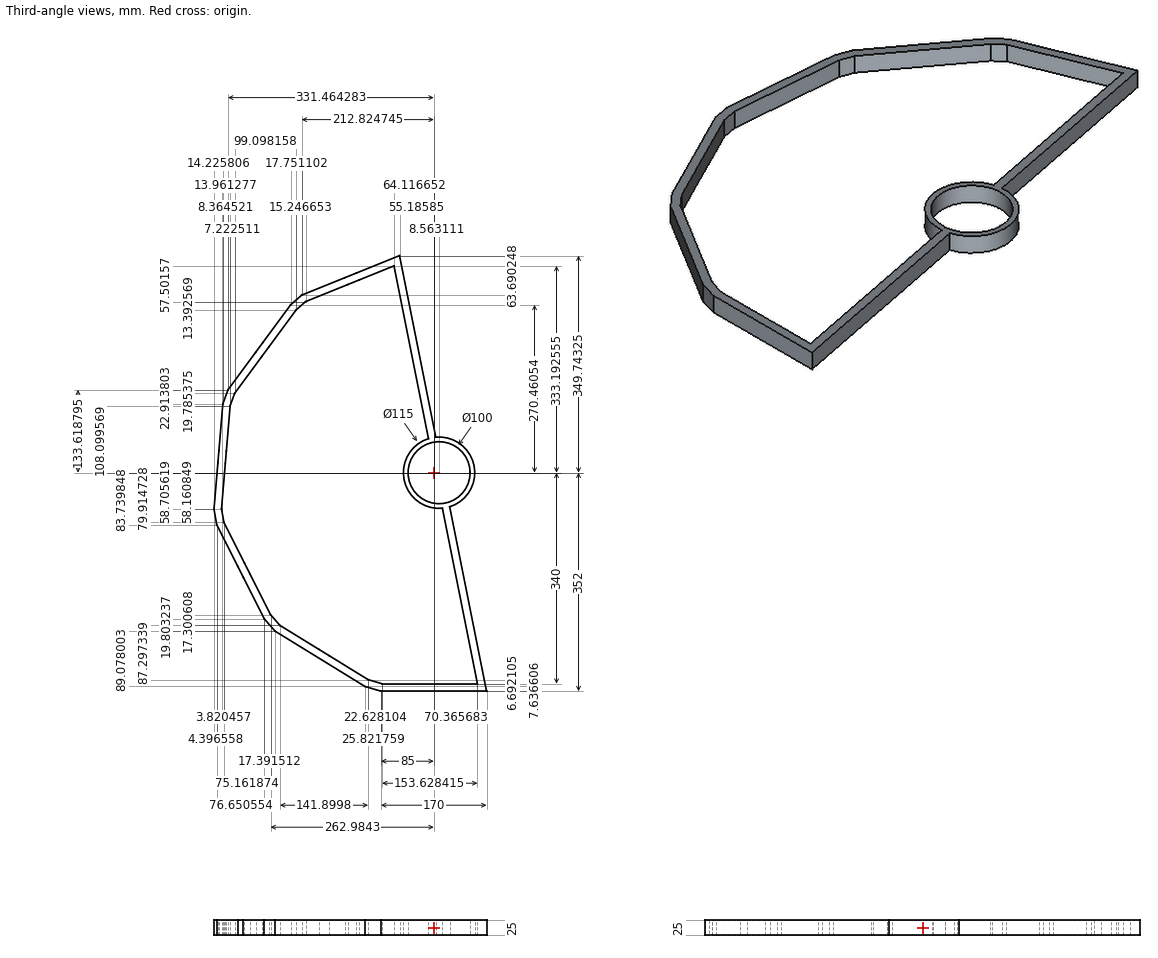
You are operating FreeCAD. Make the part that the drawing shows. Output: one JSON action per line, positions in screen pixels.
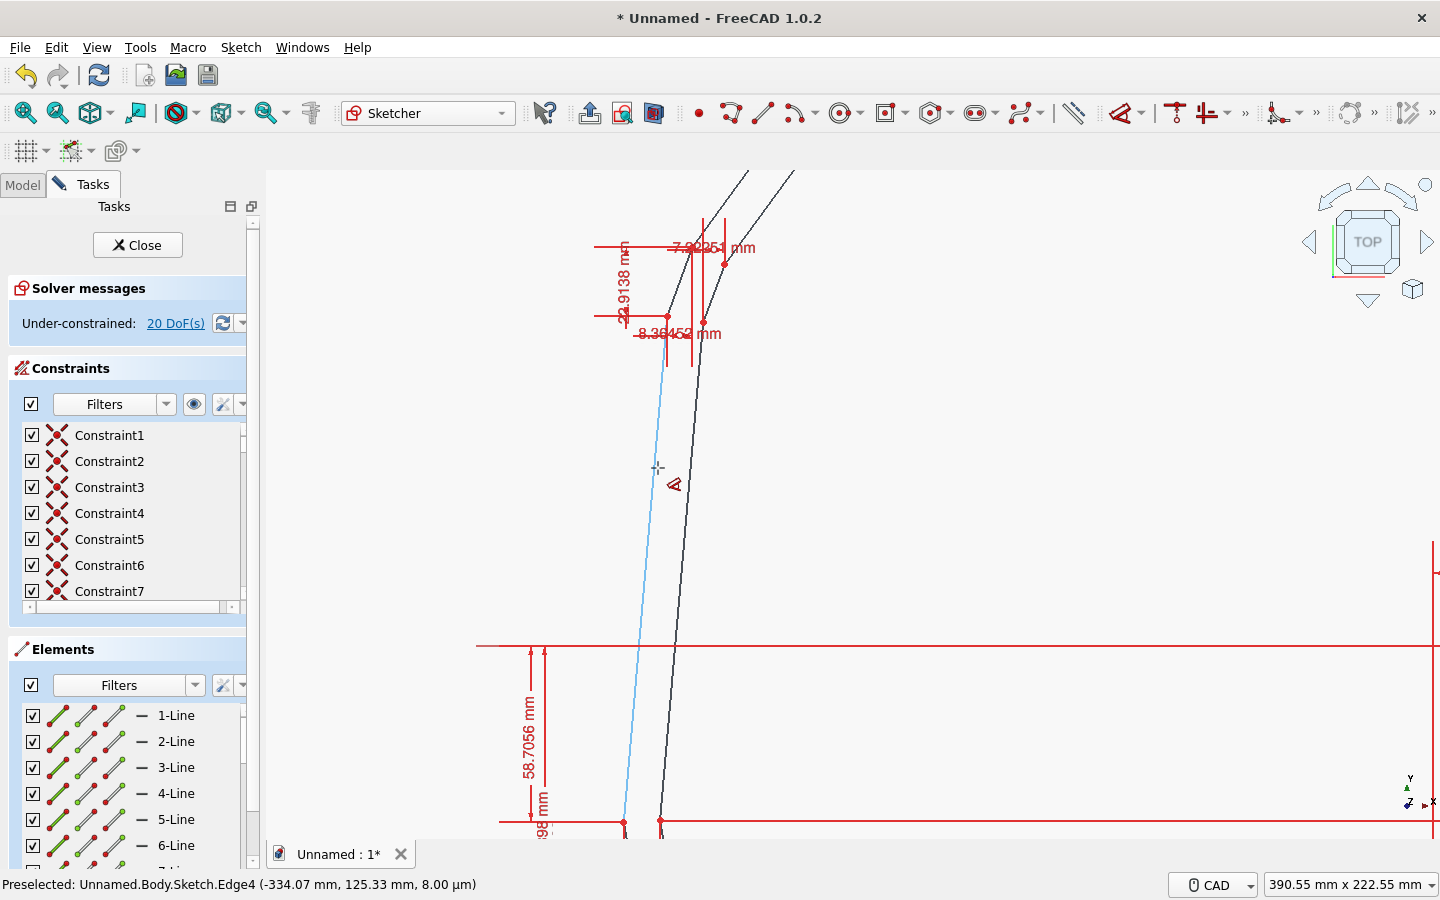
{"action": "left_click", "coordinate": [654, 468]}
{"action": "left_click", "coordinate": [636, 258]}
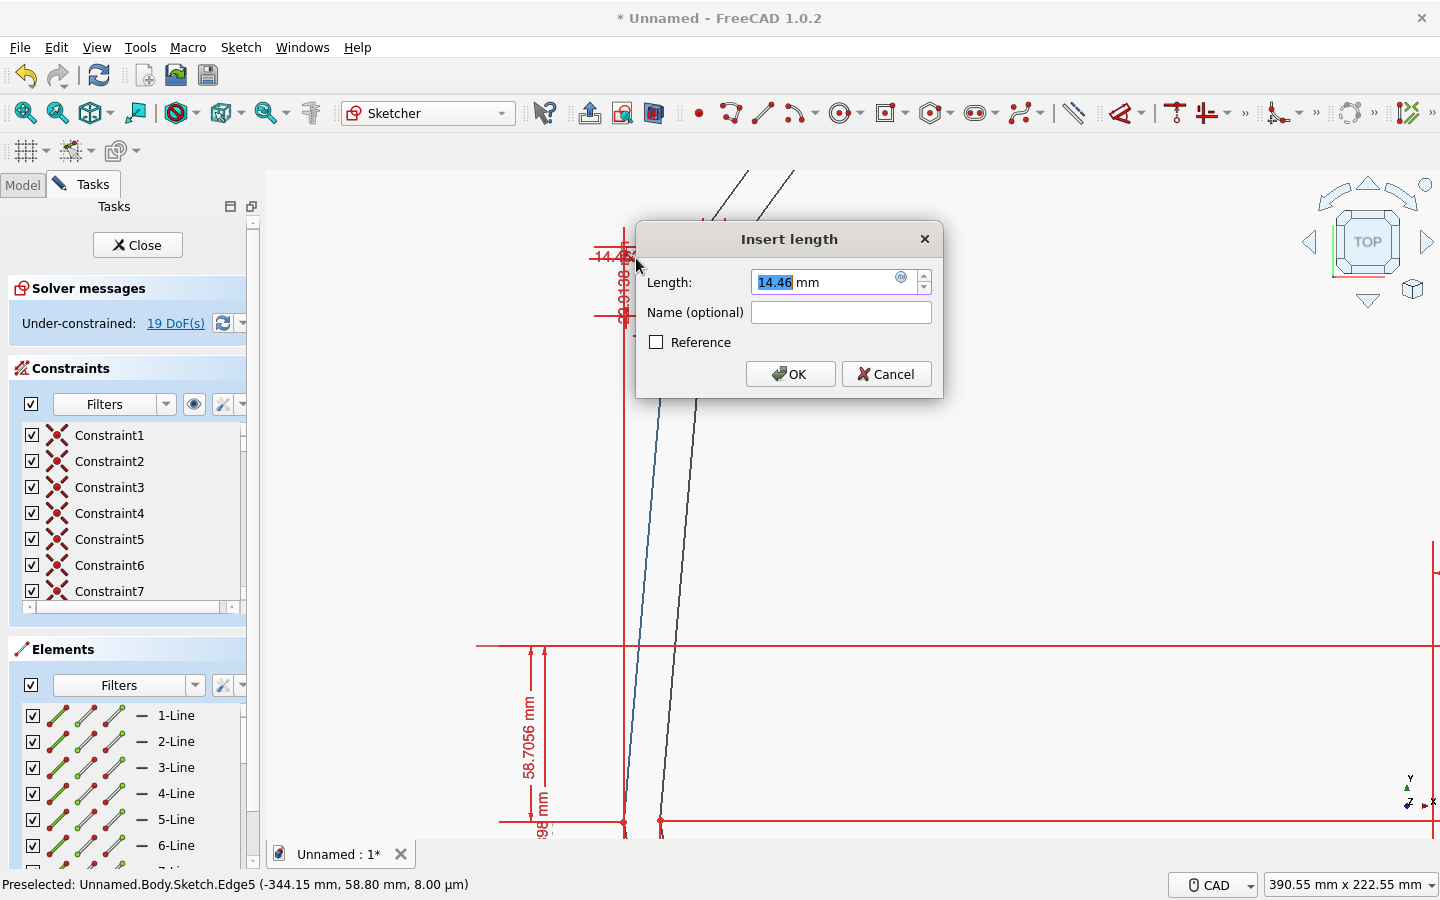
{"action": "type", "text": "14.225806"}
{"action": "key", "text": "Return"}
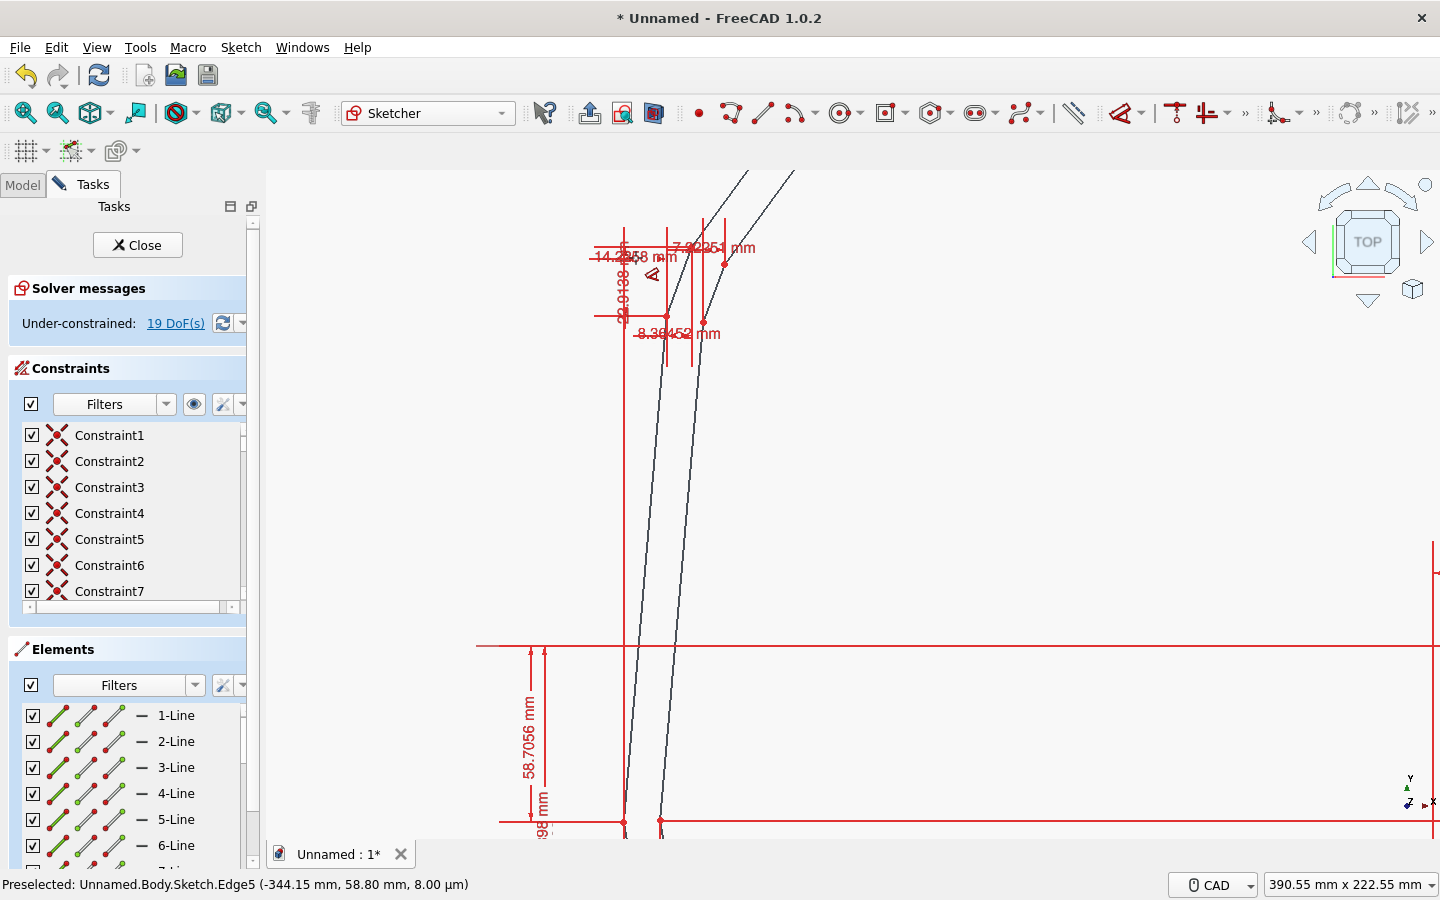
{"action": "scroll", "coordinate": [658, 468], "scroll_direction": "down", "scroll_amount": 8}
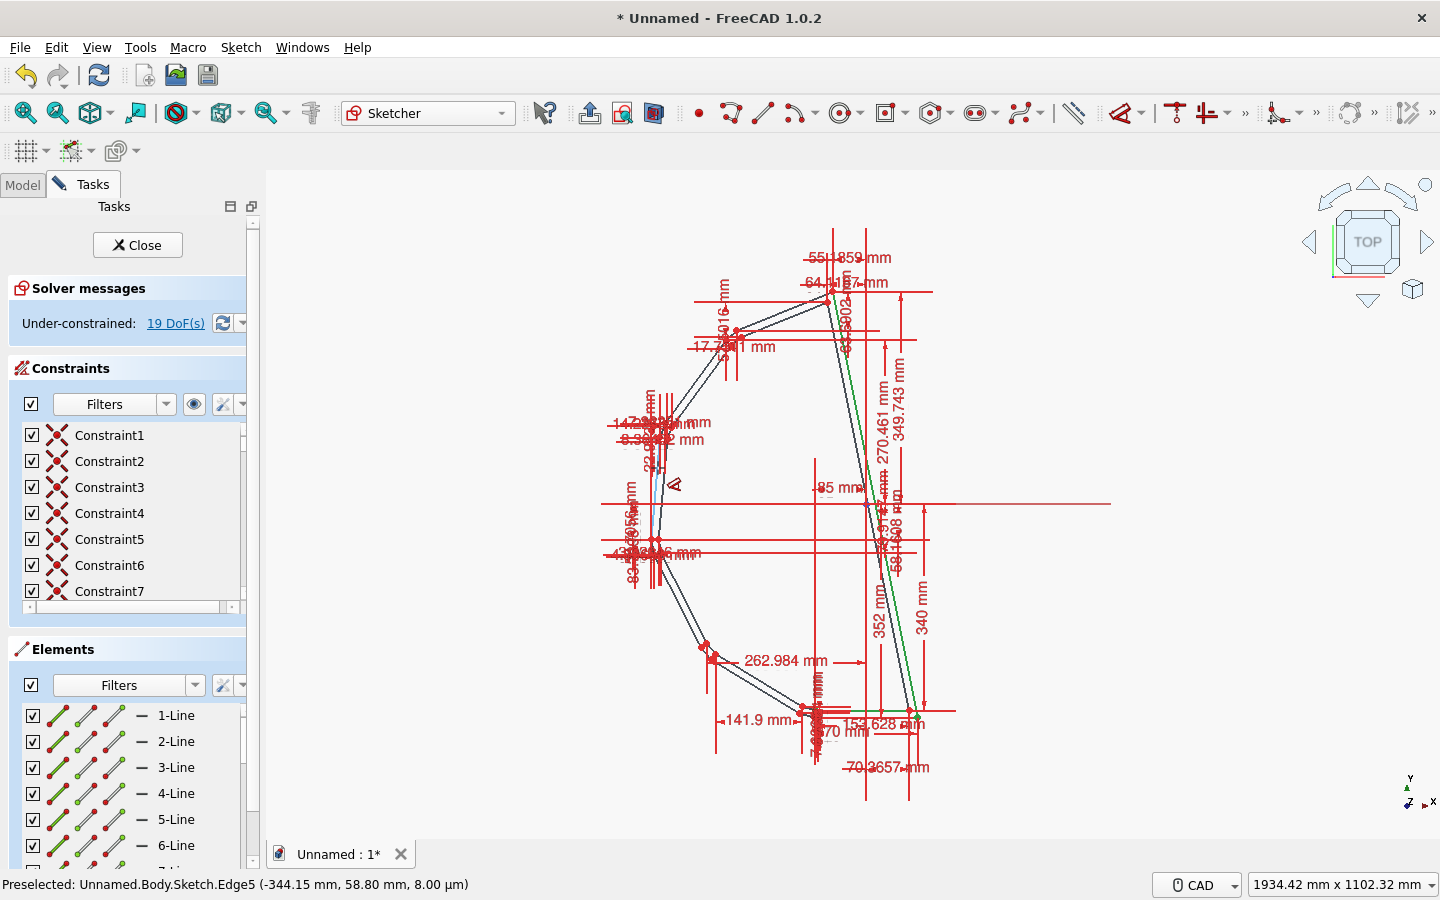
{"action": "scroll", "coordinate": [668, 583], "scroll_direction": "up", "scroll_amount": 4}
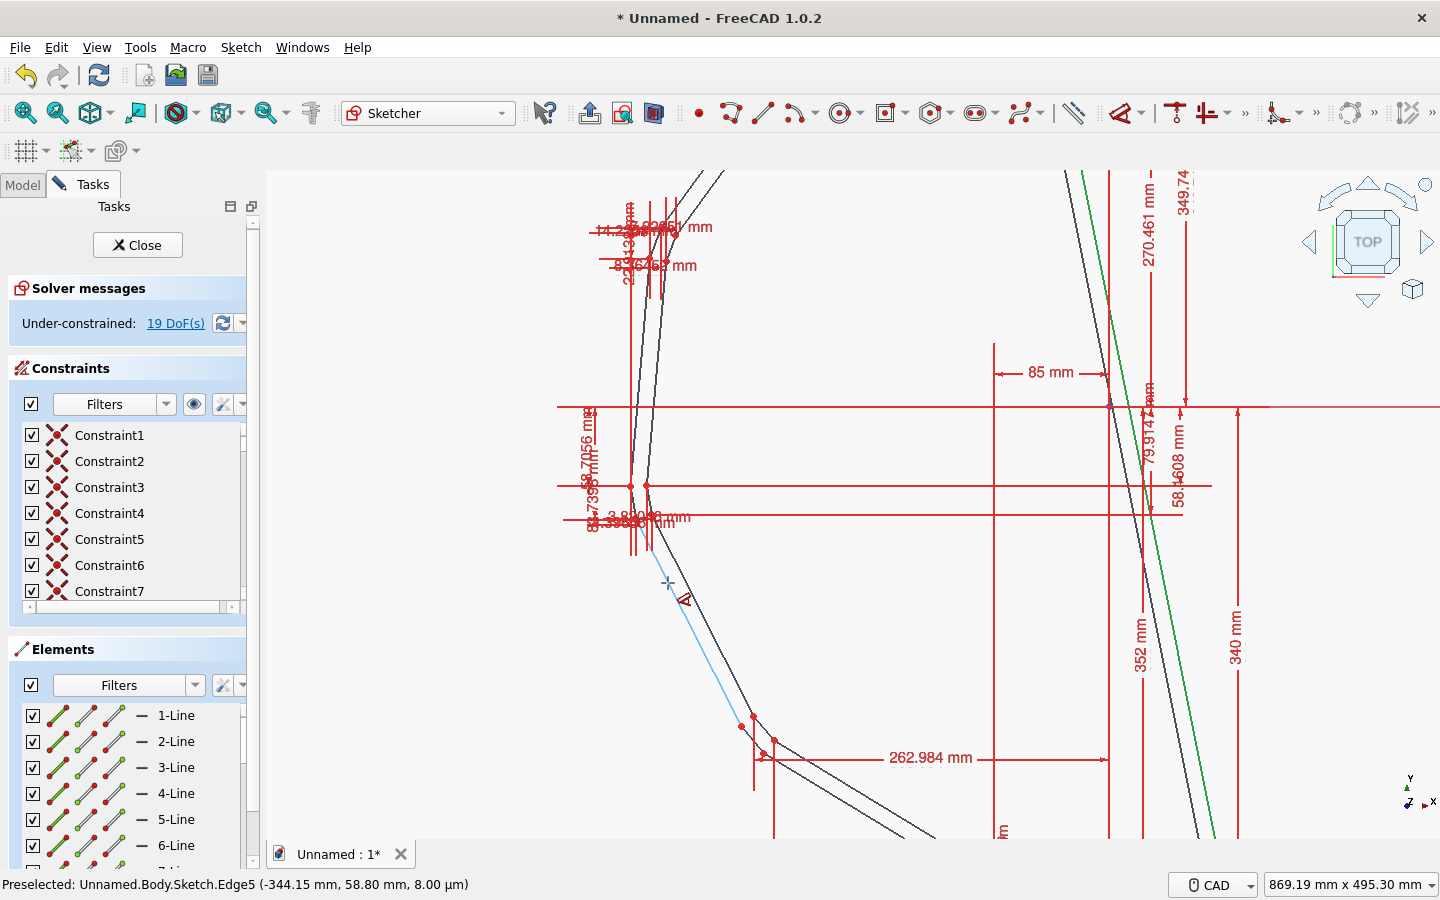
{"action": "left_click", "coordinate": [668, 582]}
{"action": "left_click", "coordinate": [689, 760]}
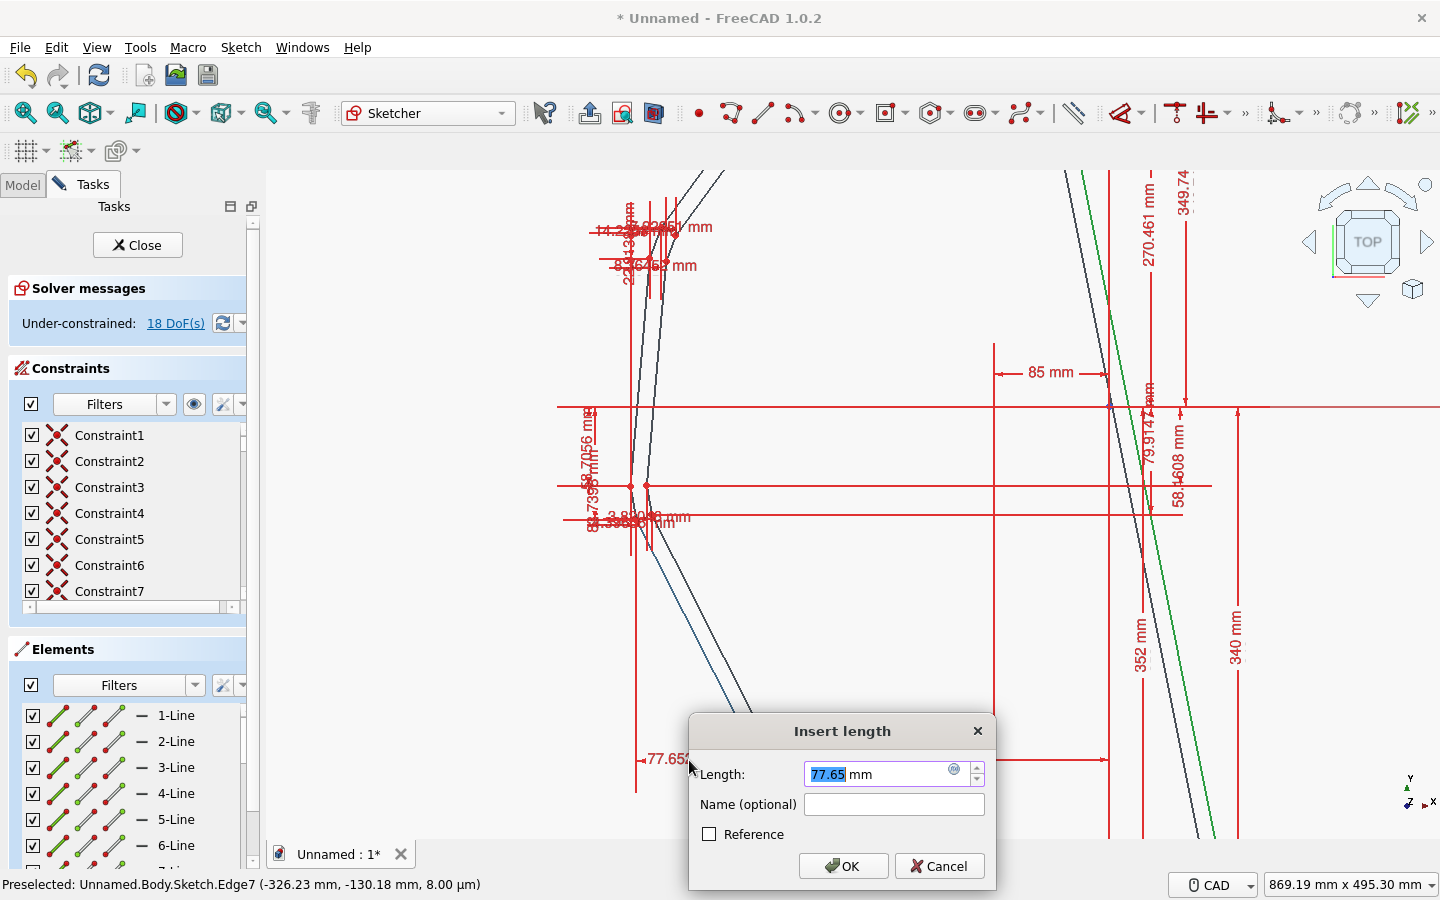
{"action": "type", "text": "76.650554"}
{"action": "key", "text": "Return"}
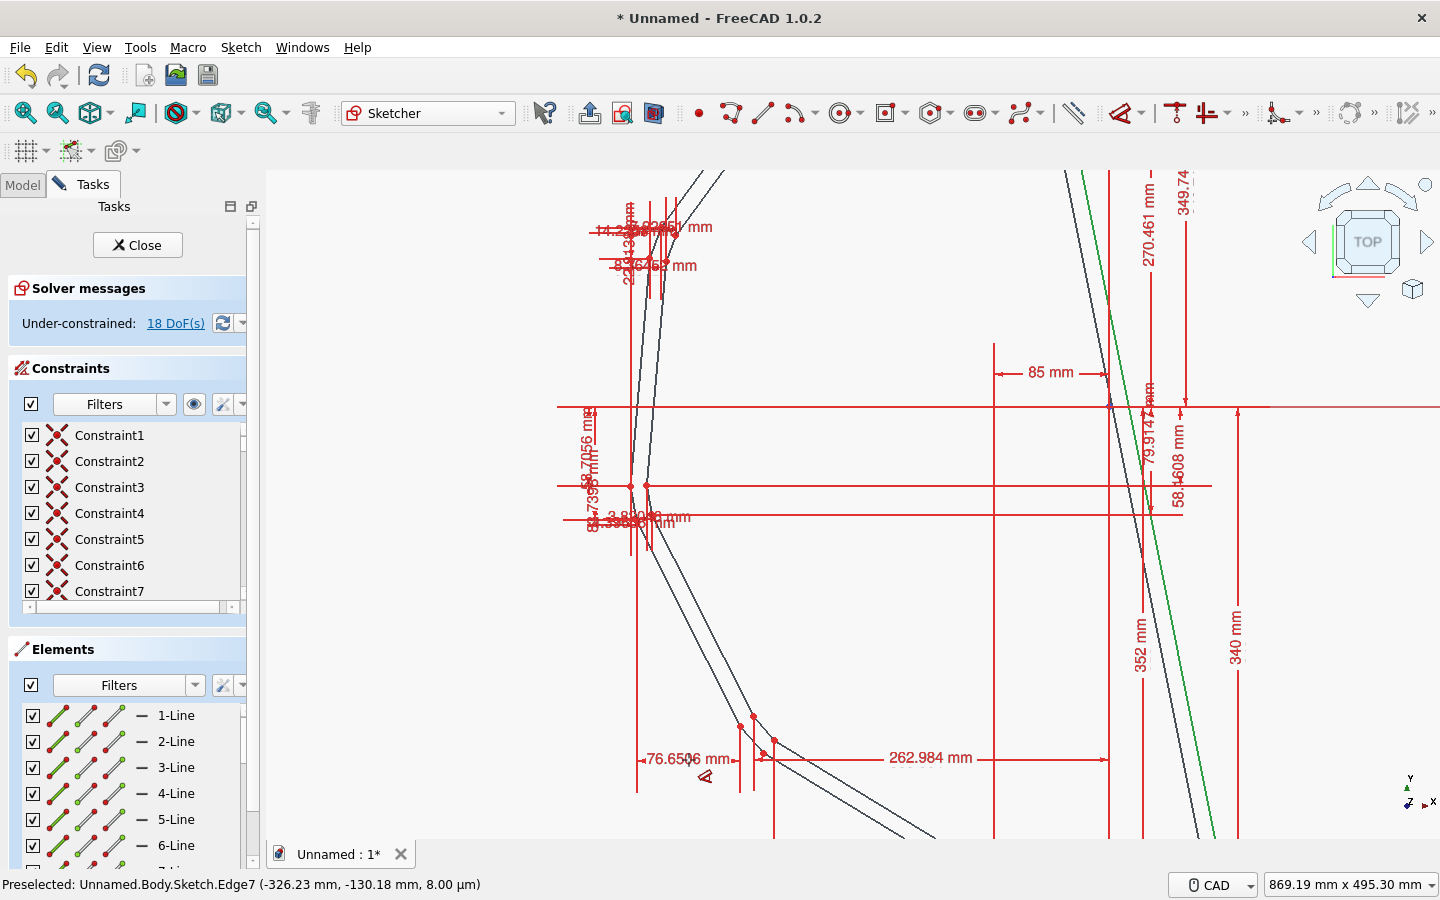
{"action": "scroll", "coordinate": [747, 734], "scroll_direction": "up", "scroll_amount": 3}